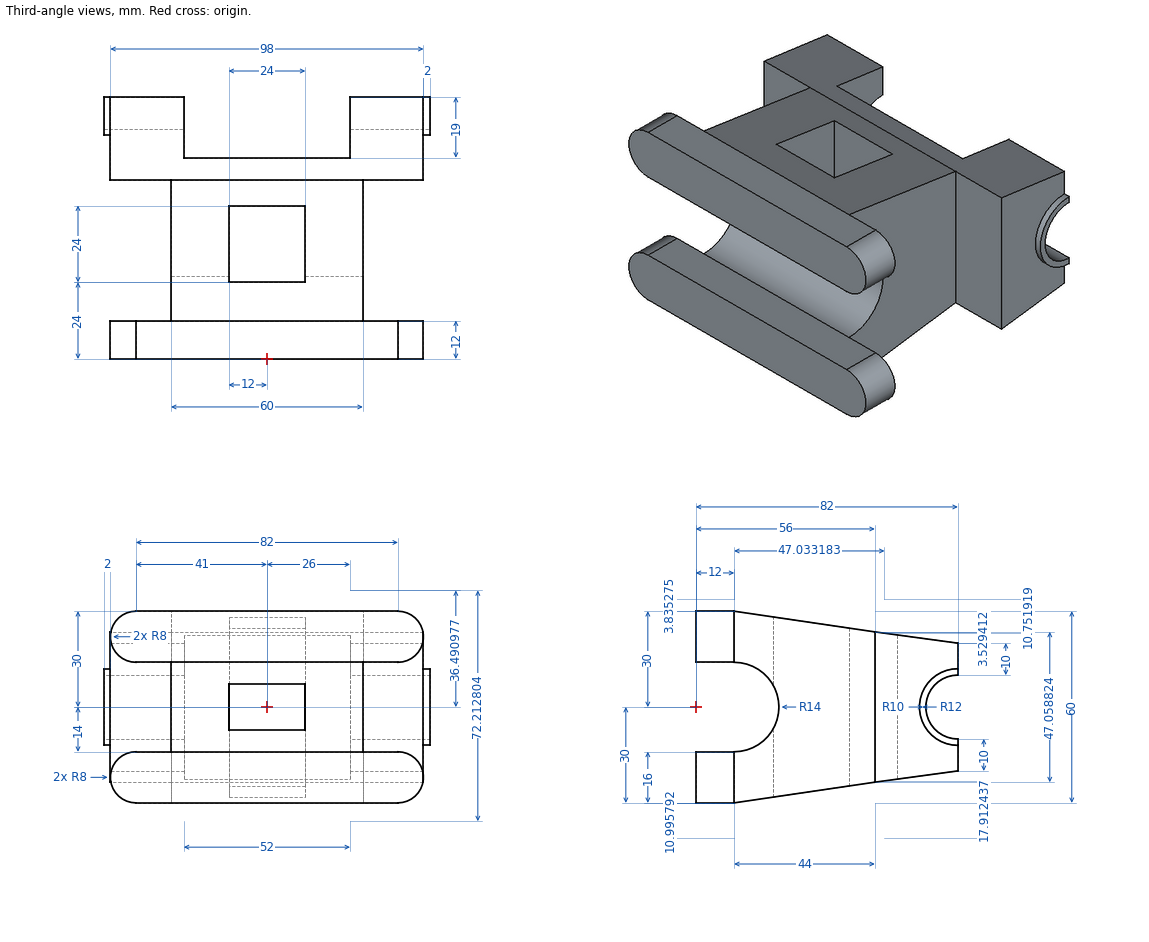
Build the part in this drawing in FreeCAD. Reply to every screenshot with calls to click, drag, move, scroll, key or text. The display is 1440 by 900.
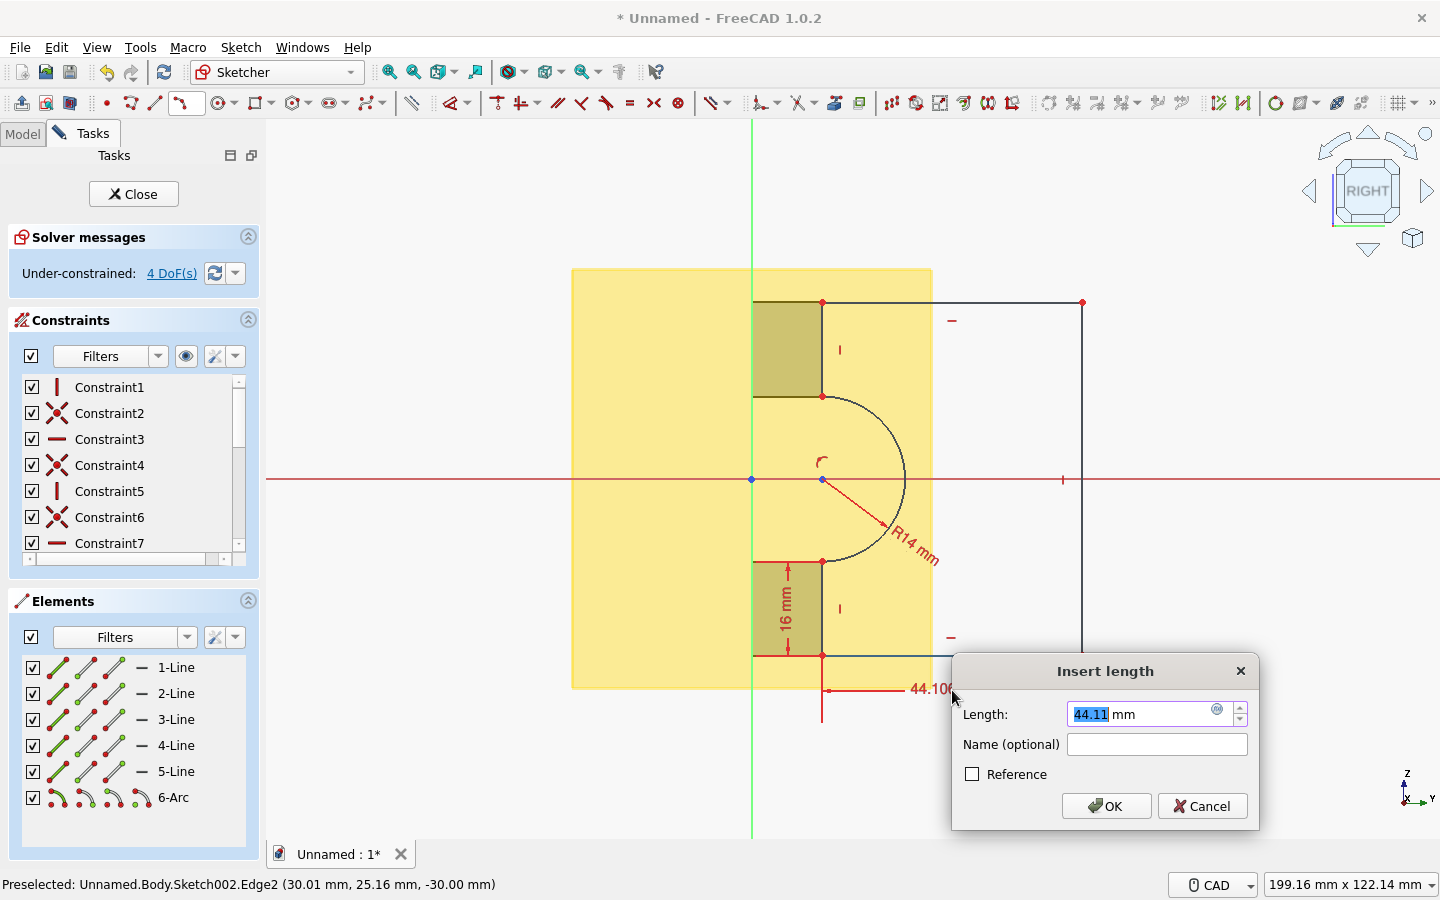
text(44)
key(Return)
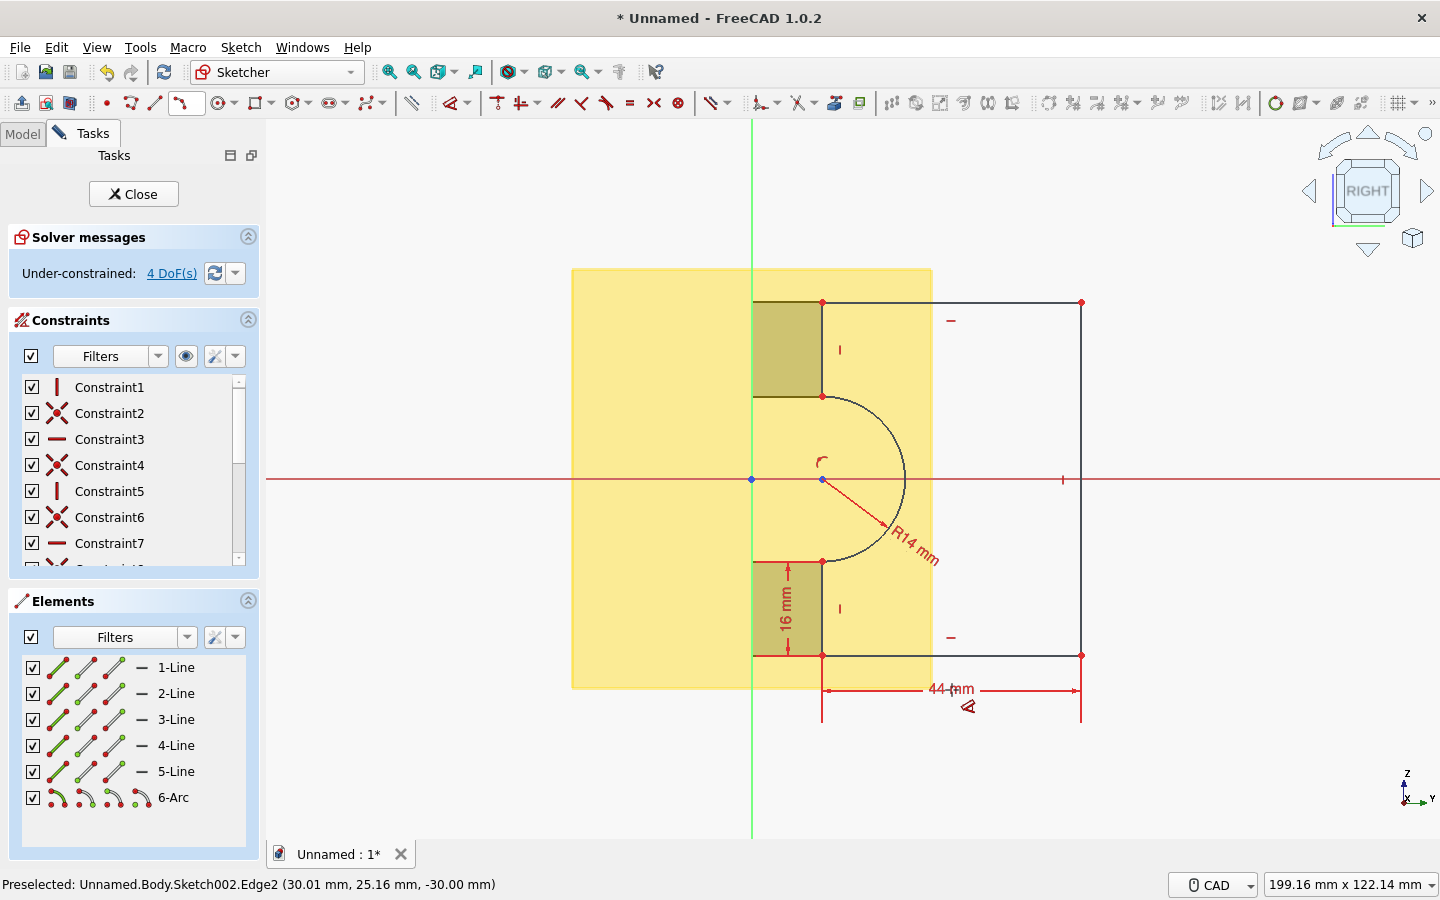
click(1081, 550)
click(1115, 398)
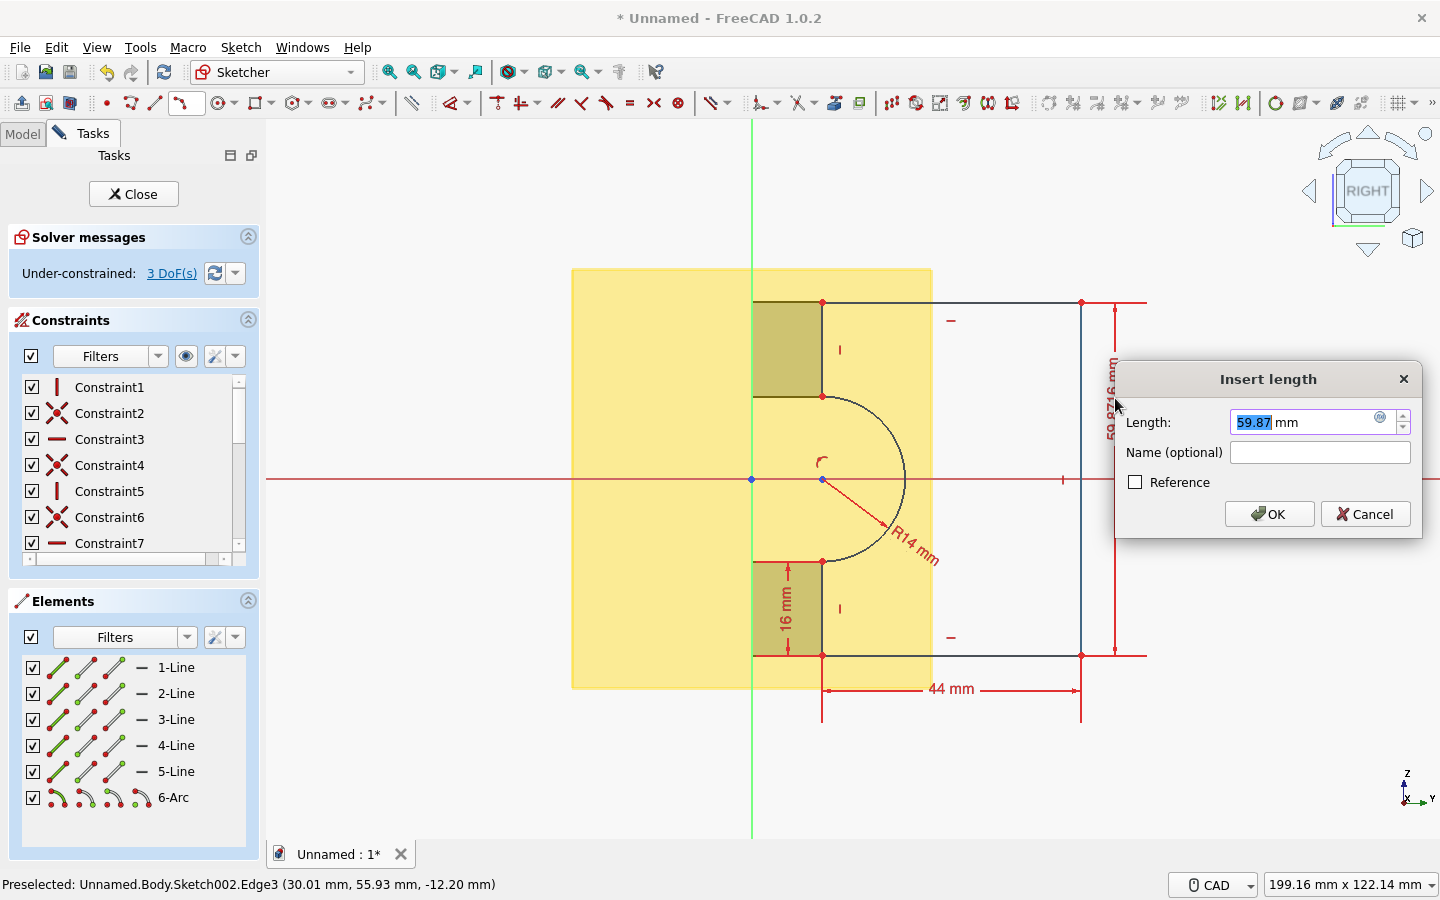
text(60)
key(Return)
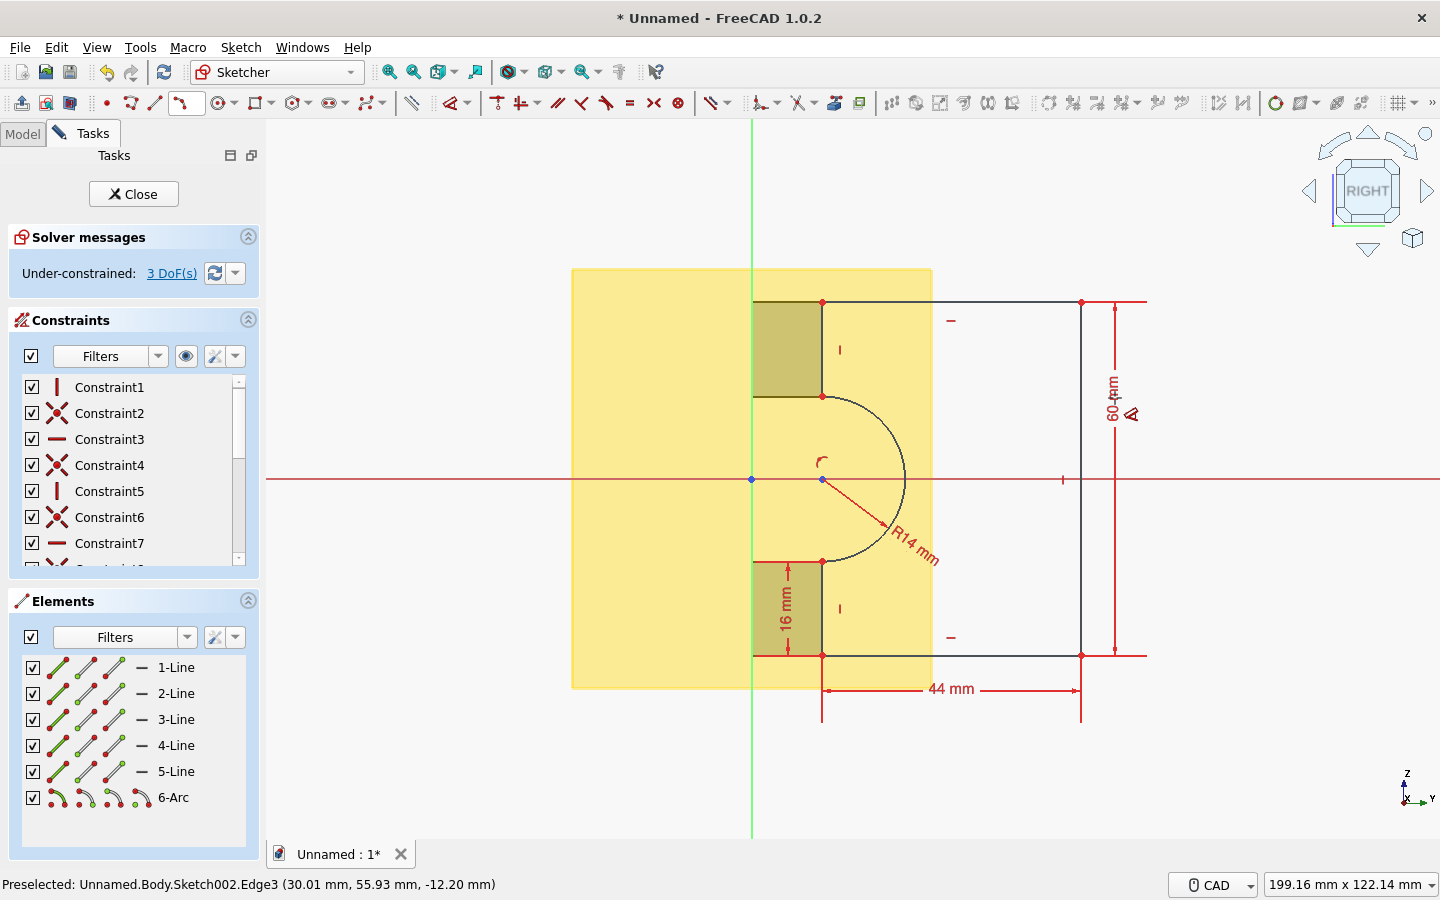
click(1004, 302)
click(952, 268)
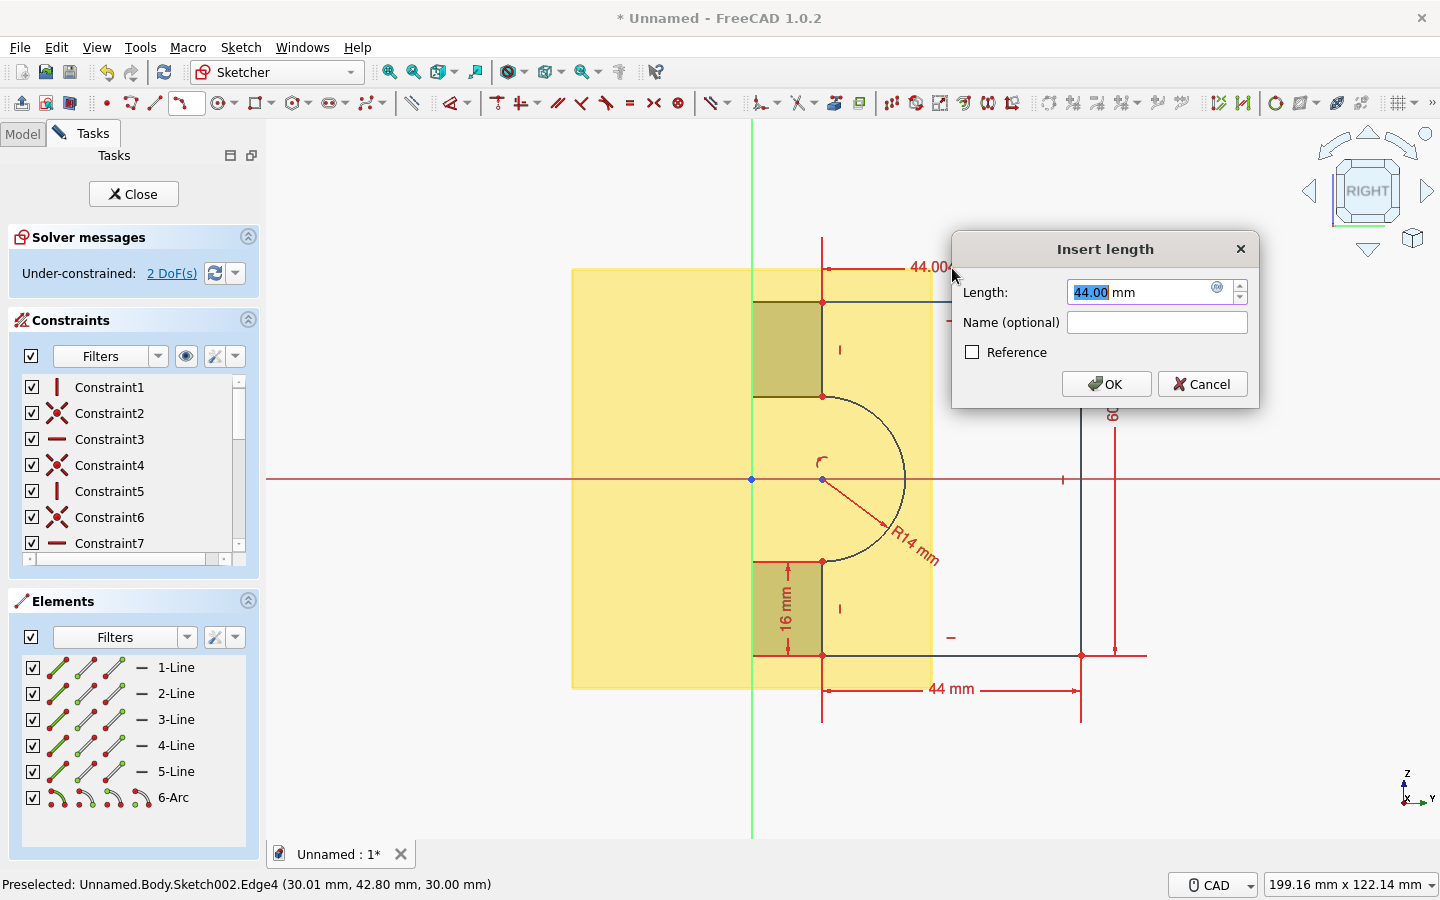
text(44)
key(Return)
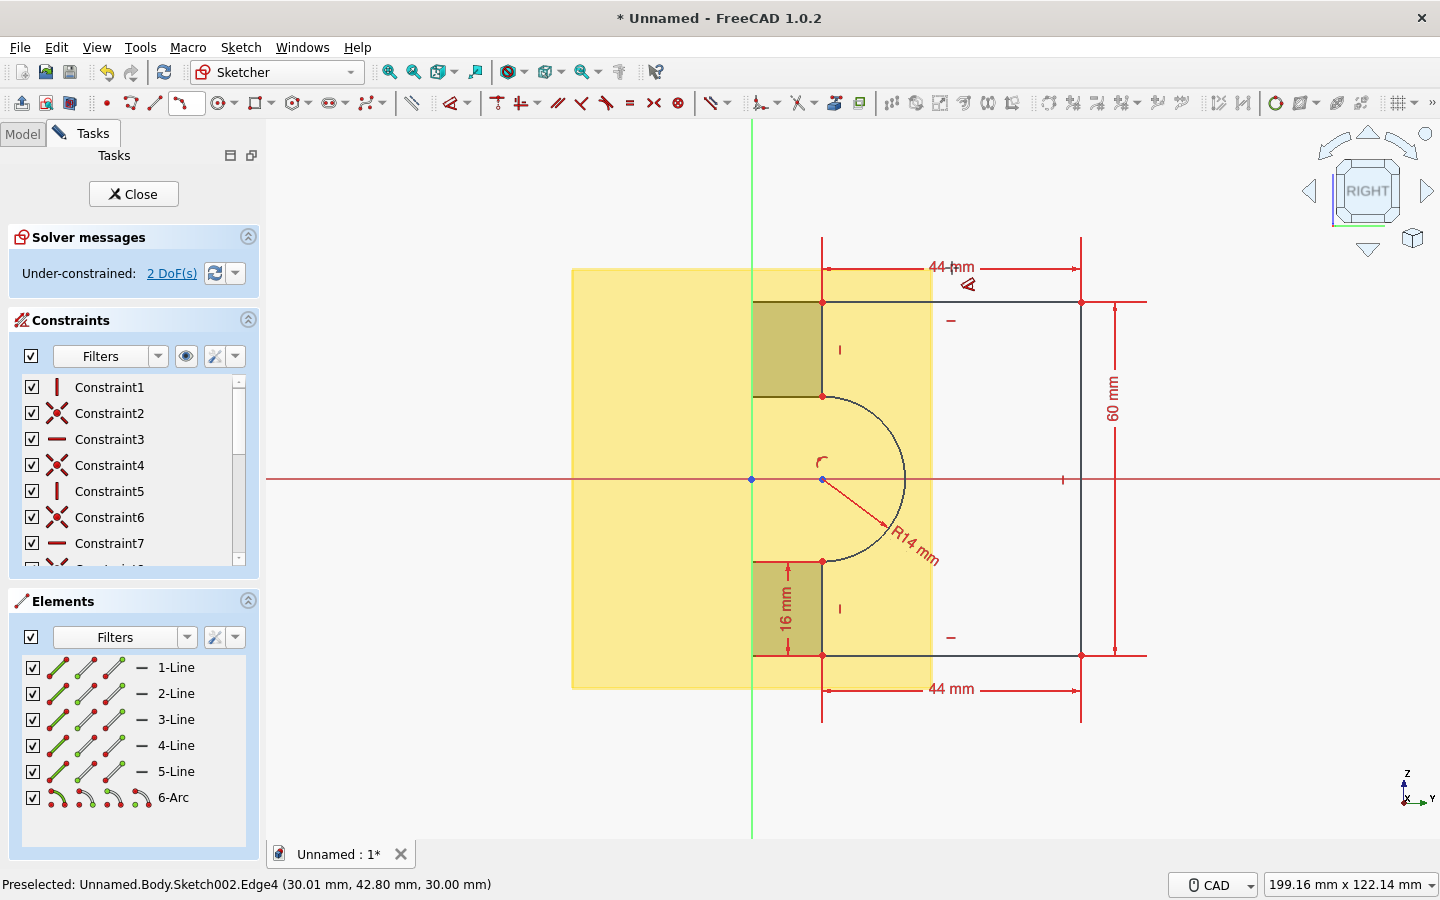
click(822, 562)
click(787, 445)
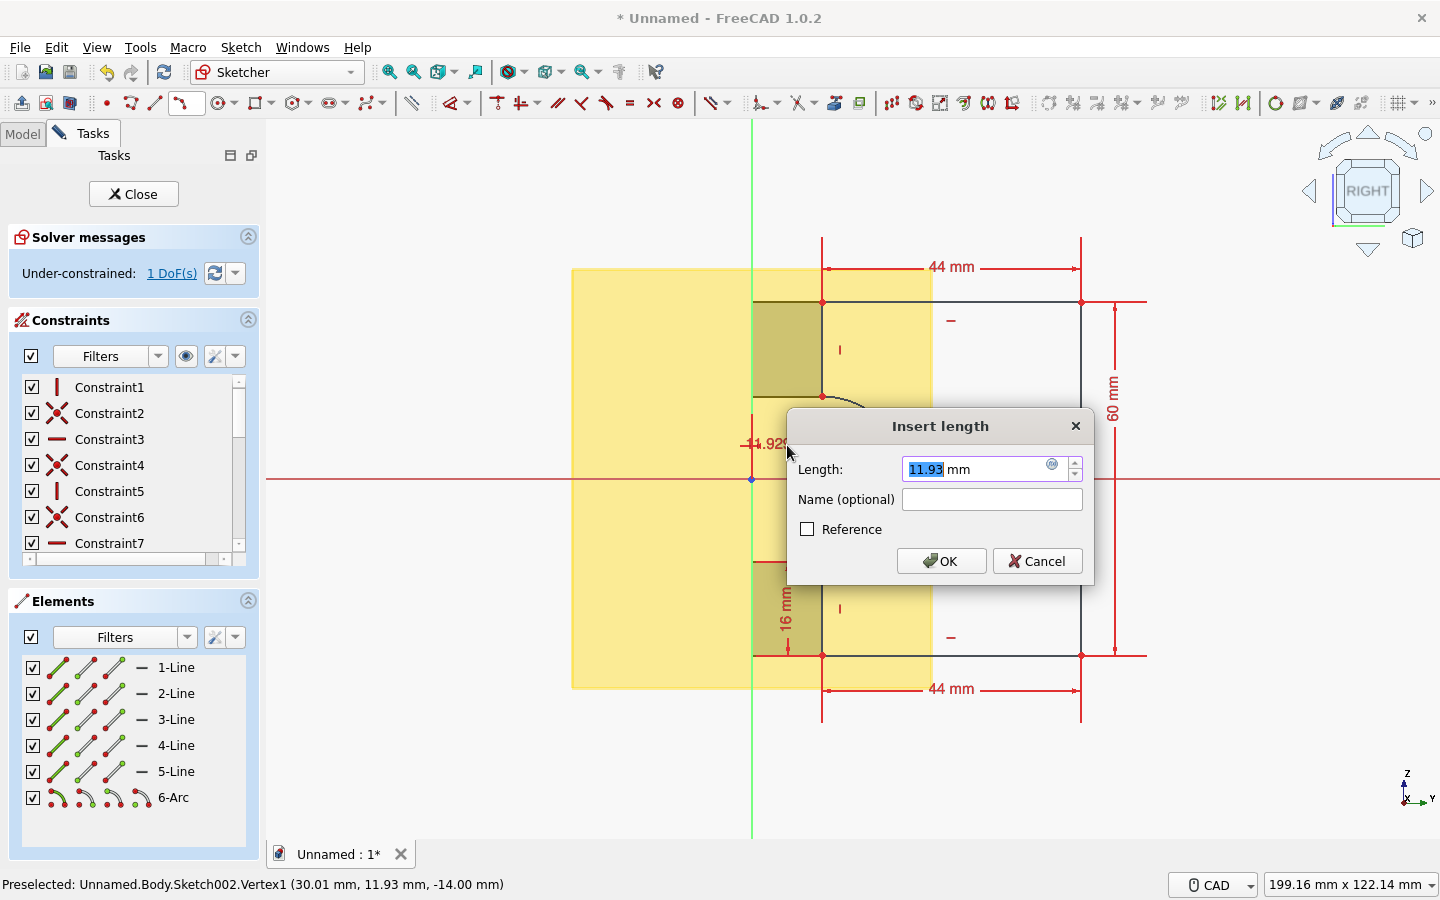
text(12)
key(Return)